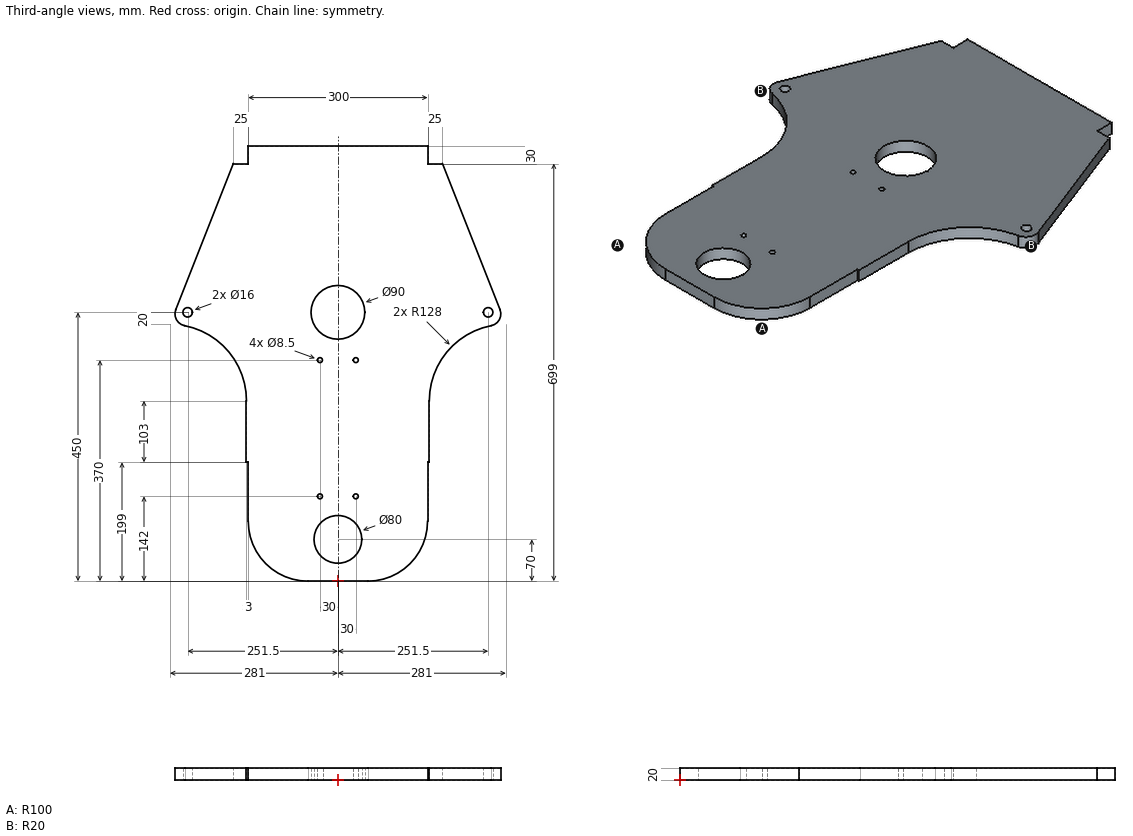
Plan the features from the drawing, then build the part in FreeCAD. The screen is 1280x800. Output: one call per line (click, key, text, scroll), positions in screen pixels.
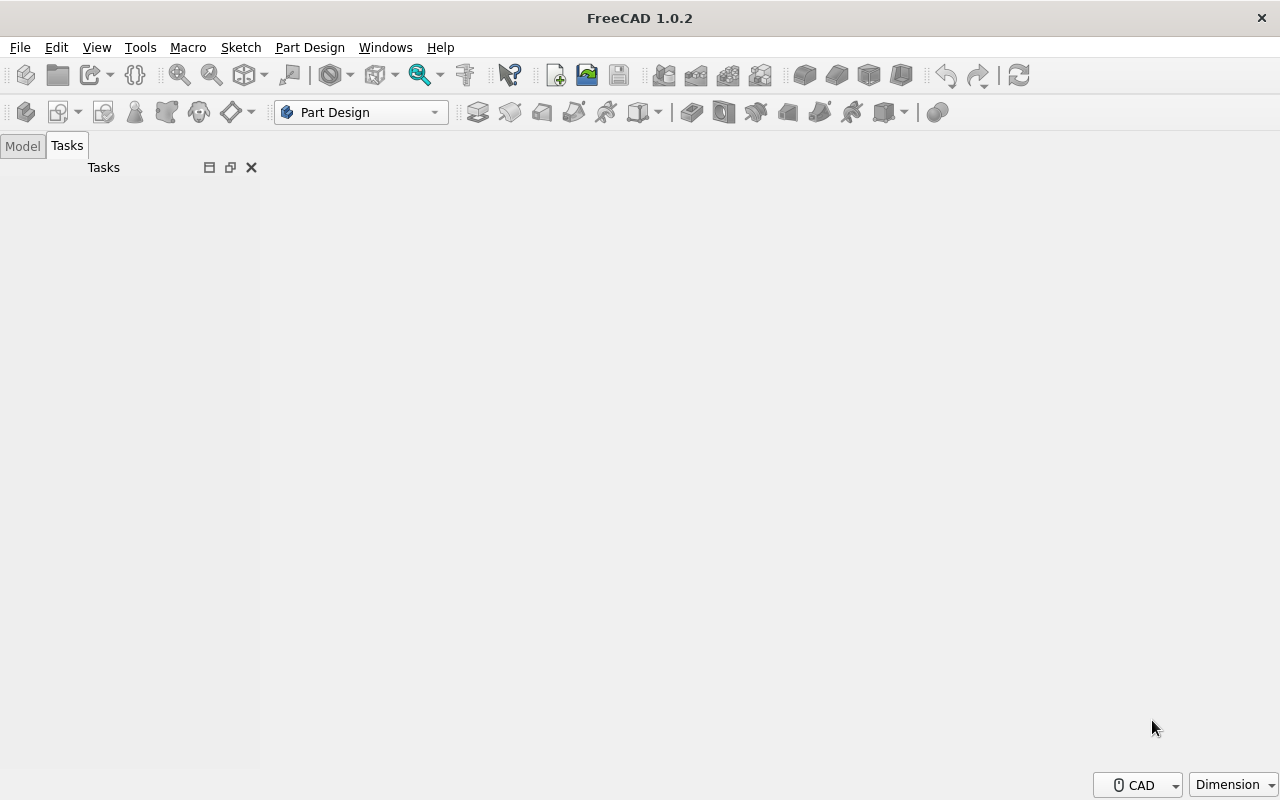
key(ctrl+n)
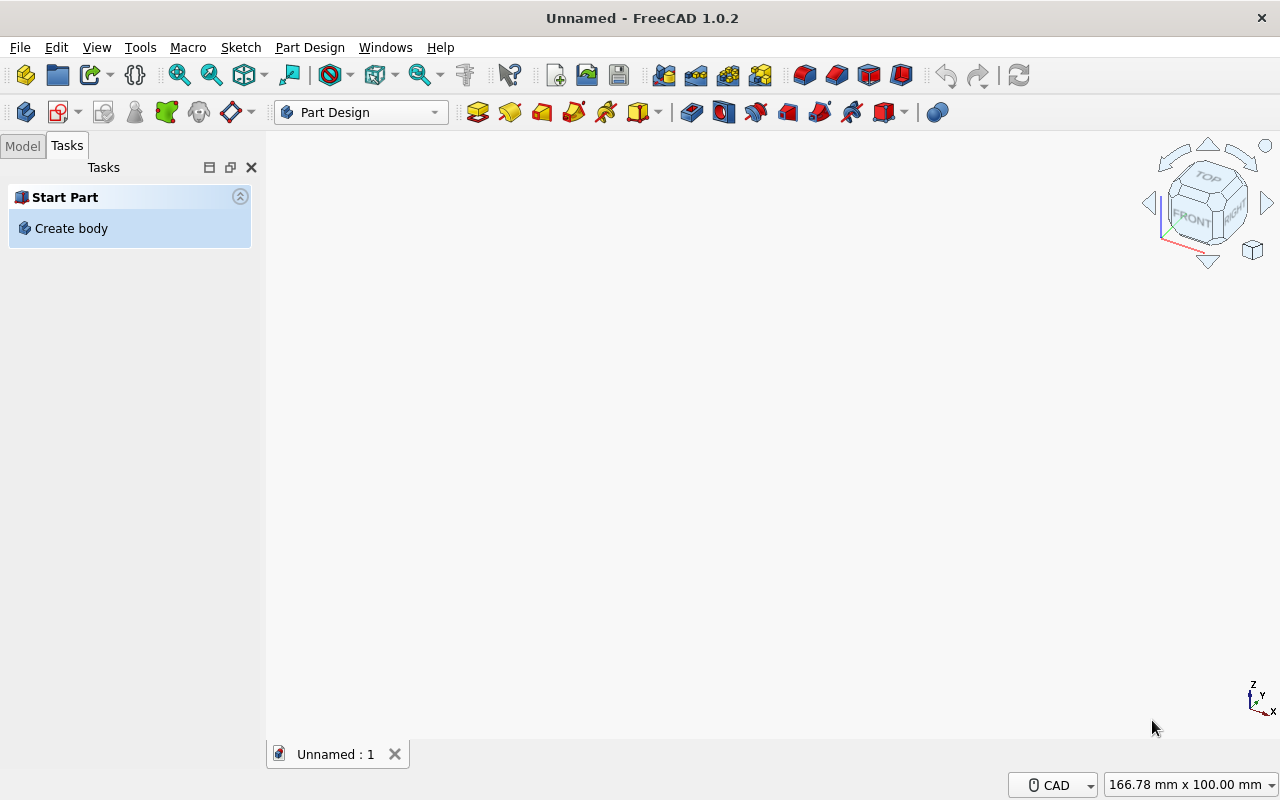
click(58, 112)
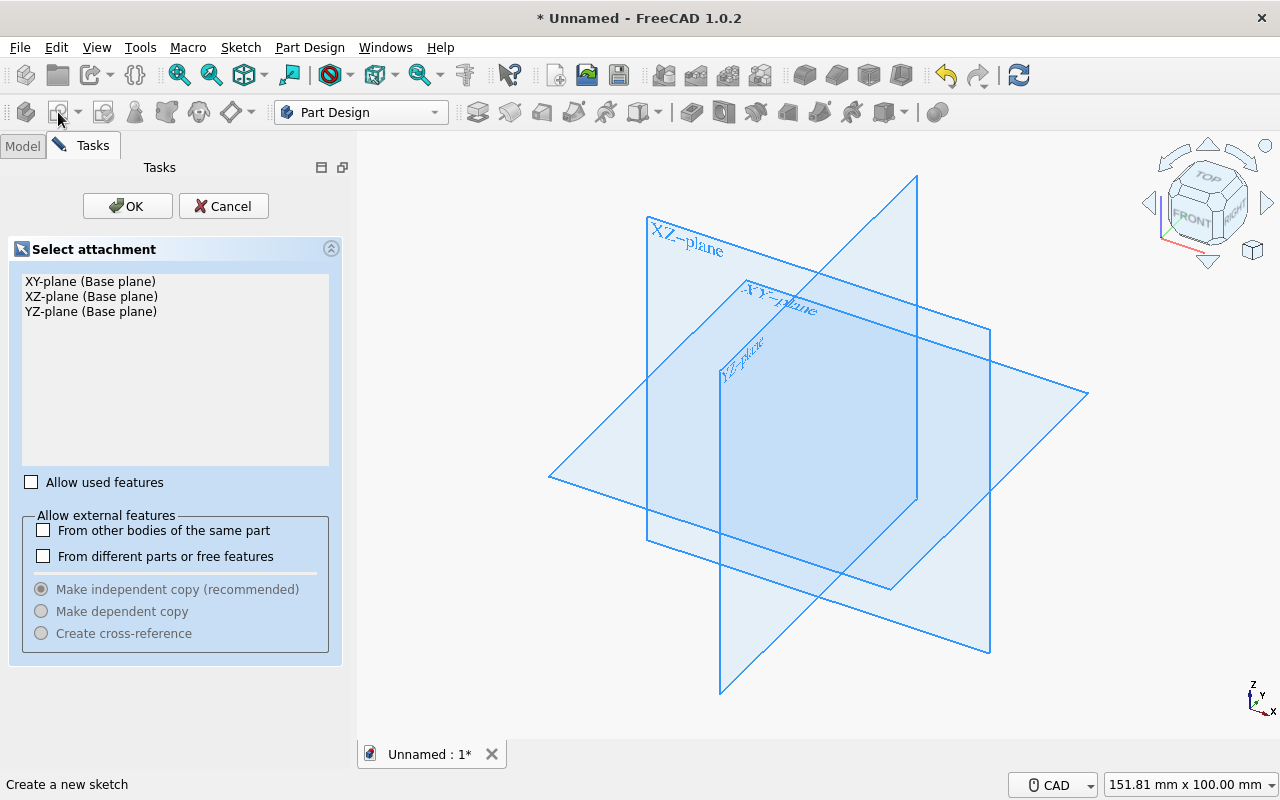
click(82, 282)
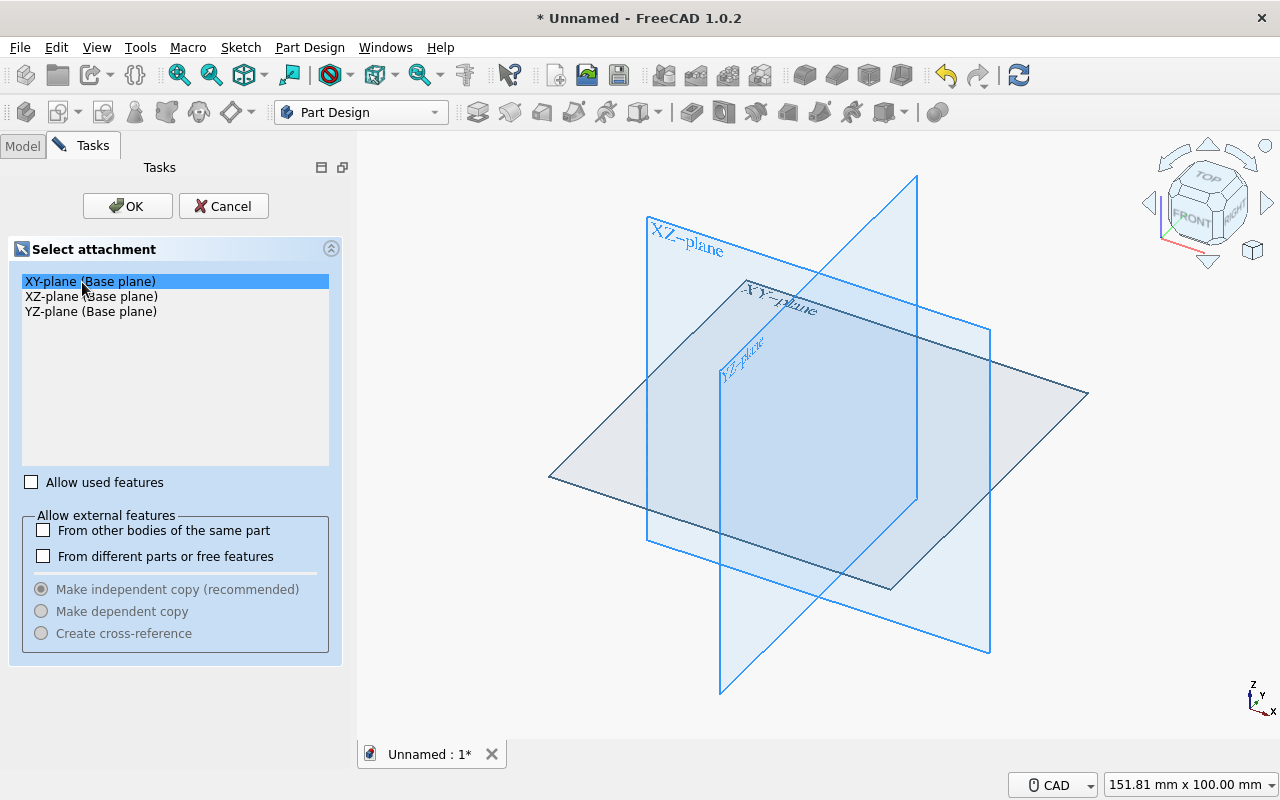
click(128, 206)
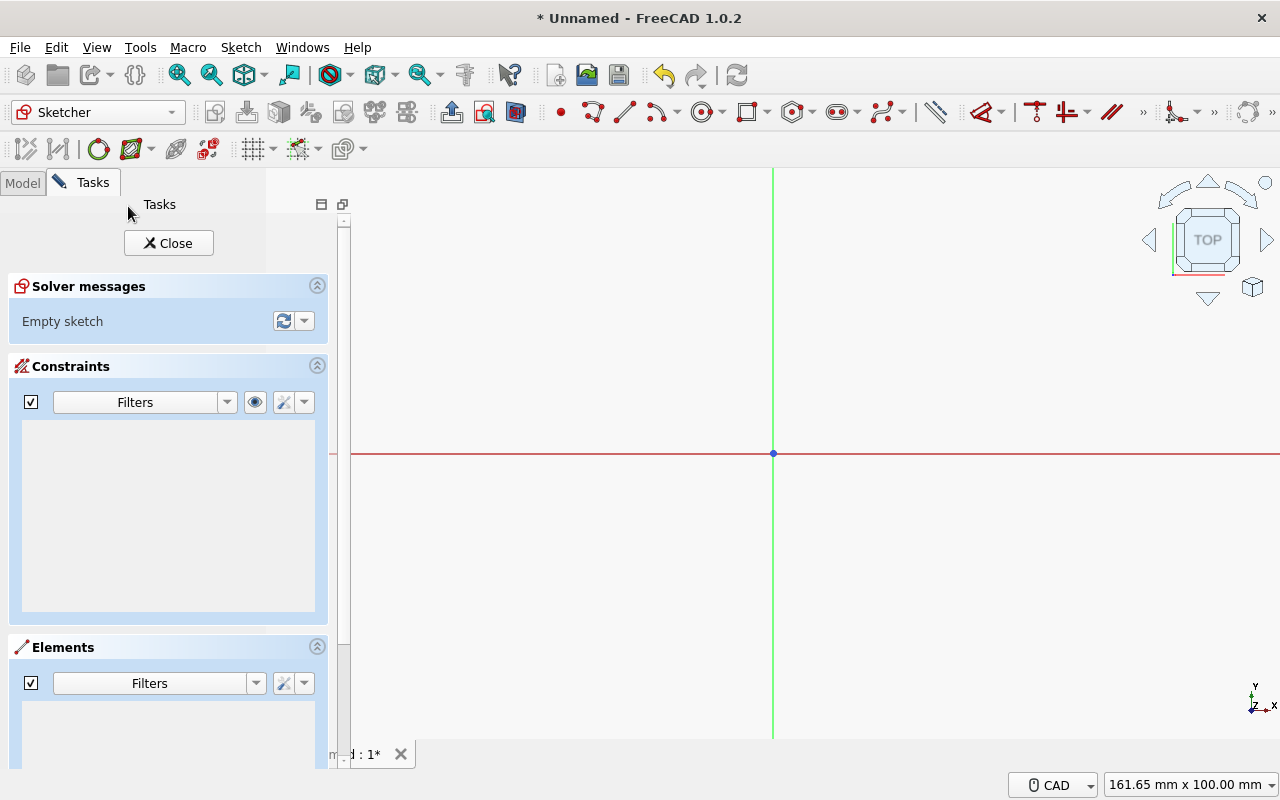
scroll(698, 661, down, 12)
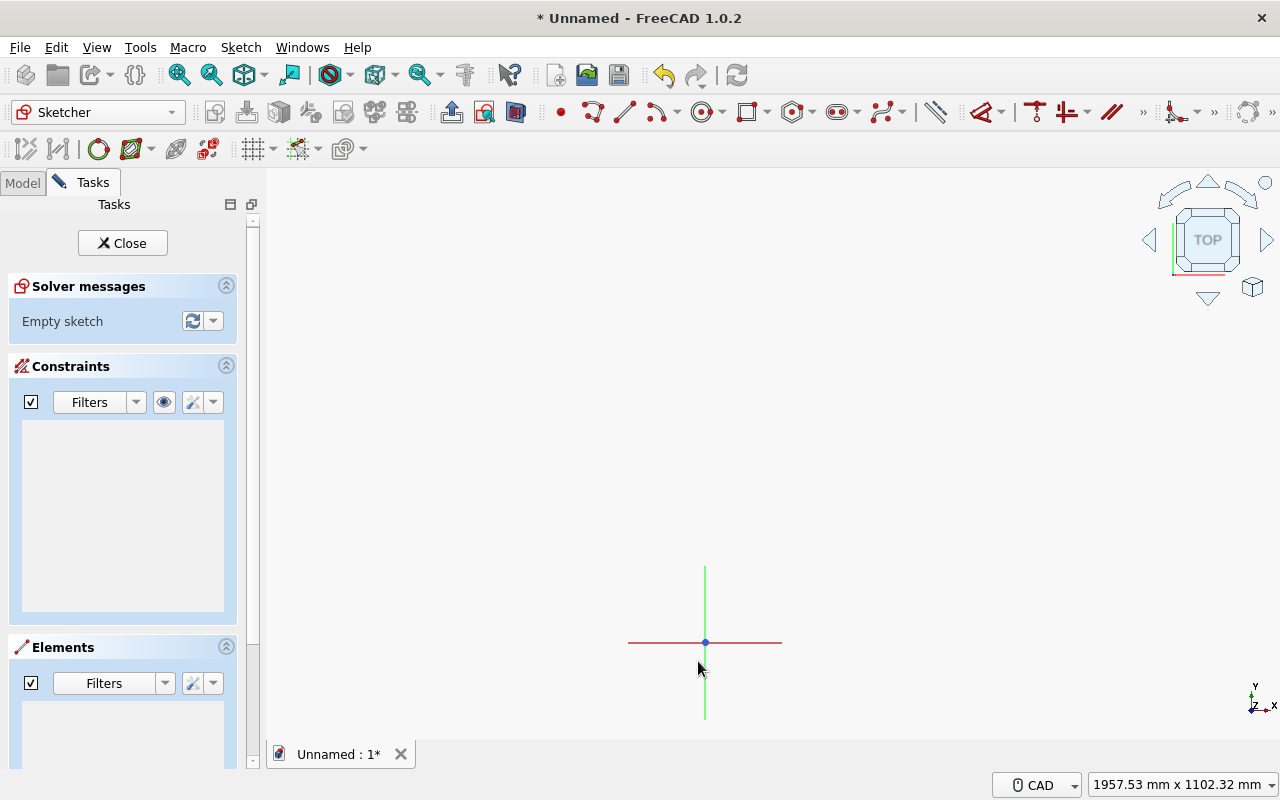
click(594, 112)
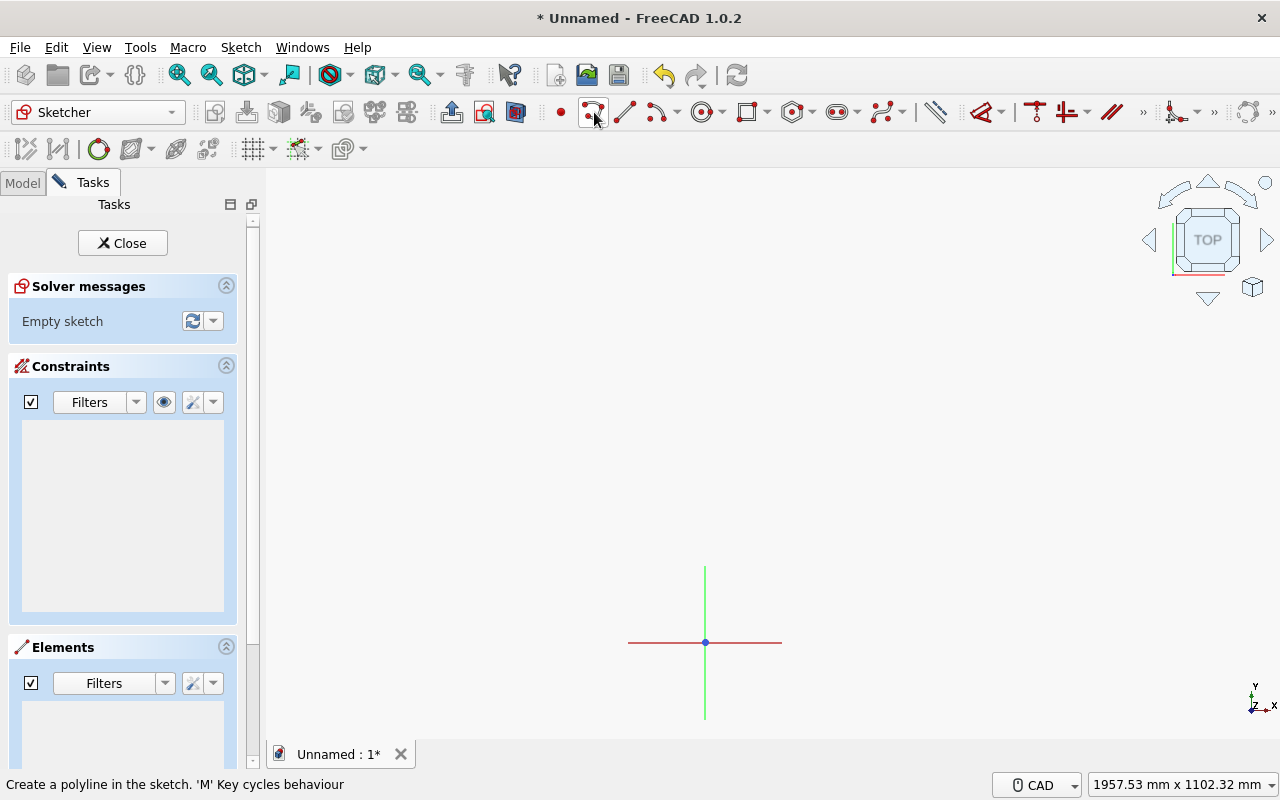
click(851, 420)
click(796, 281)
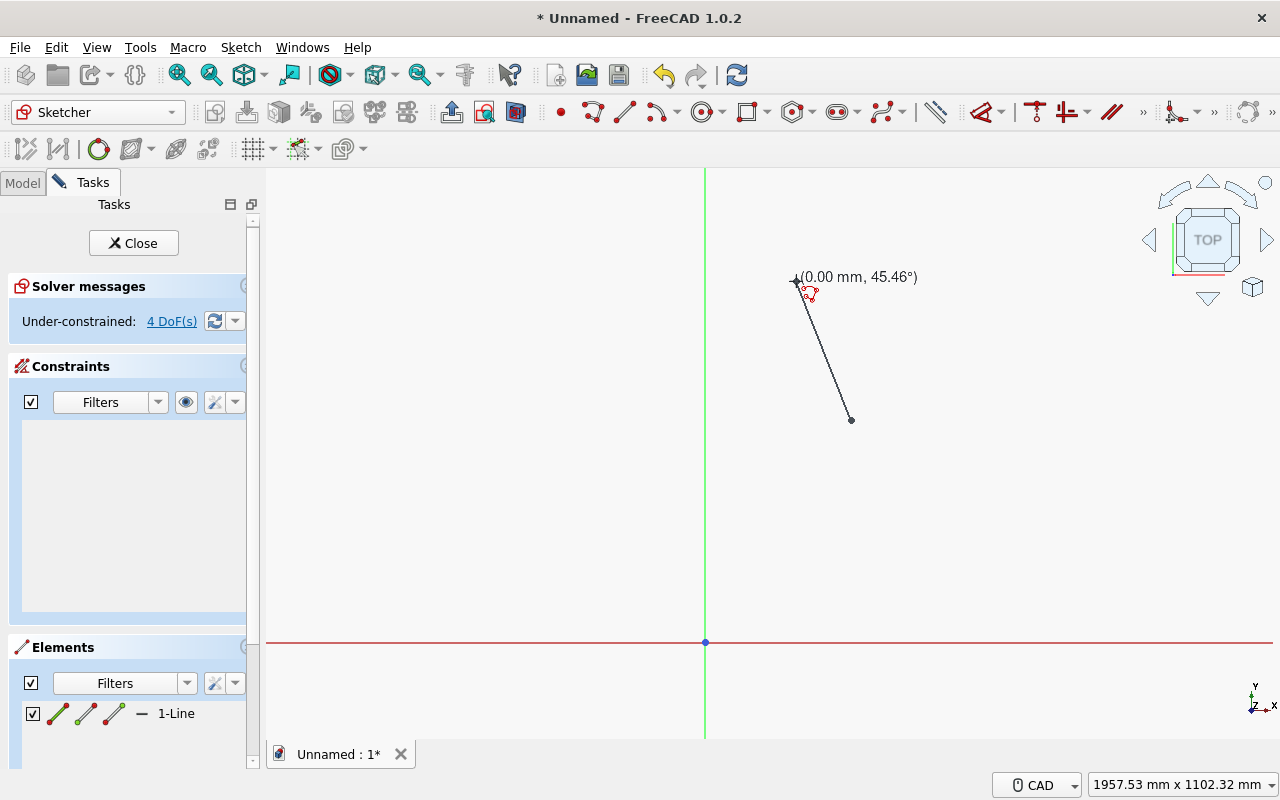
scroll(783, 281, up, 2)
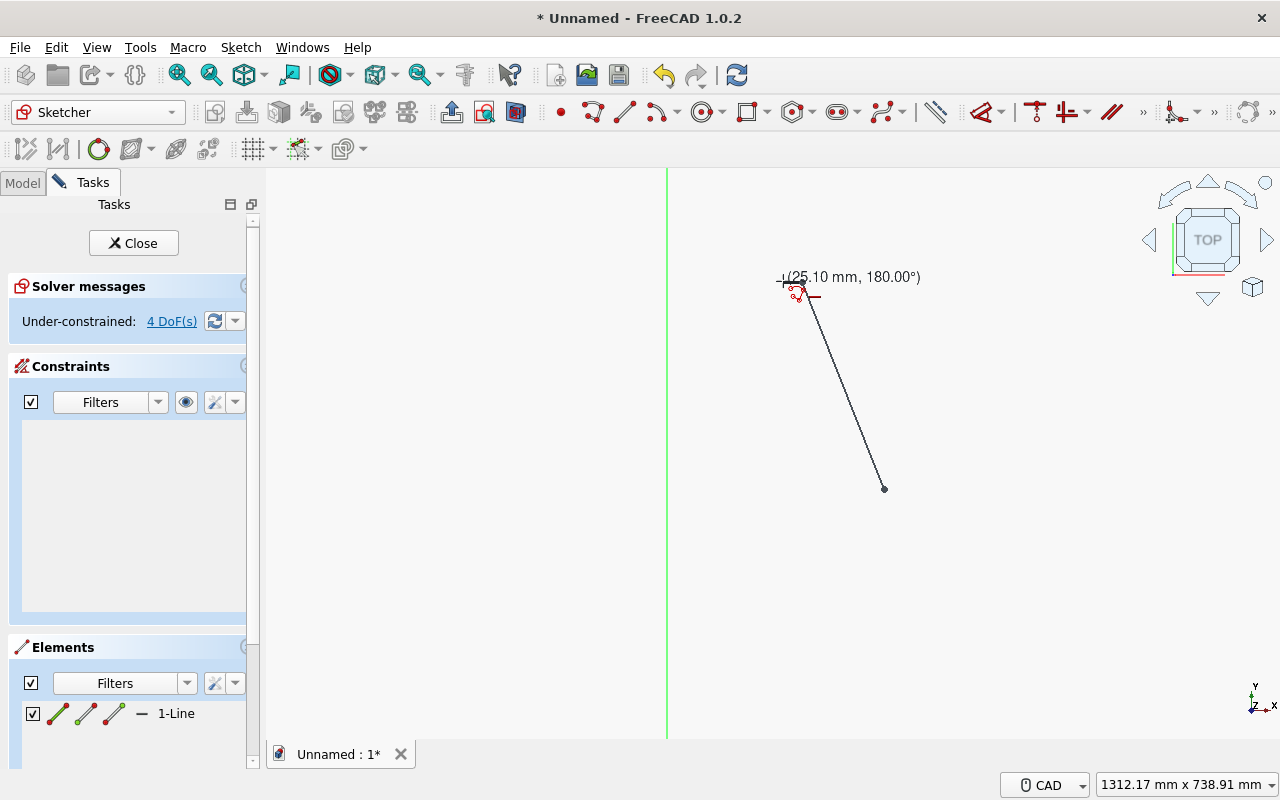
click(783, 281)
click(783, 258)
click(551, 258)
click(551, 281)
click(531, 281)
click(450, 489)
right_click(450, 489)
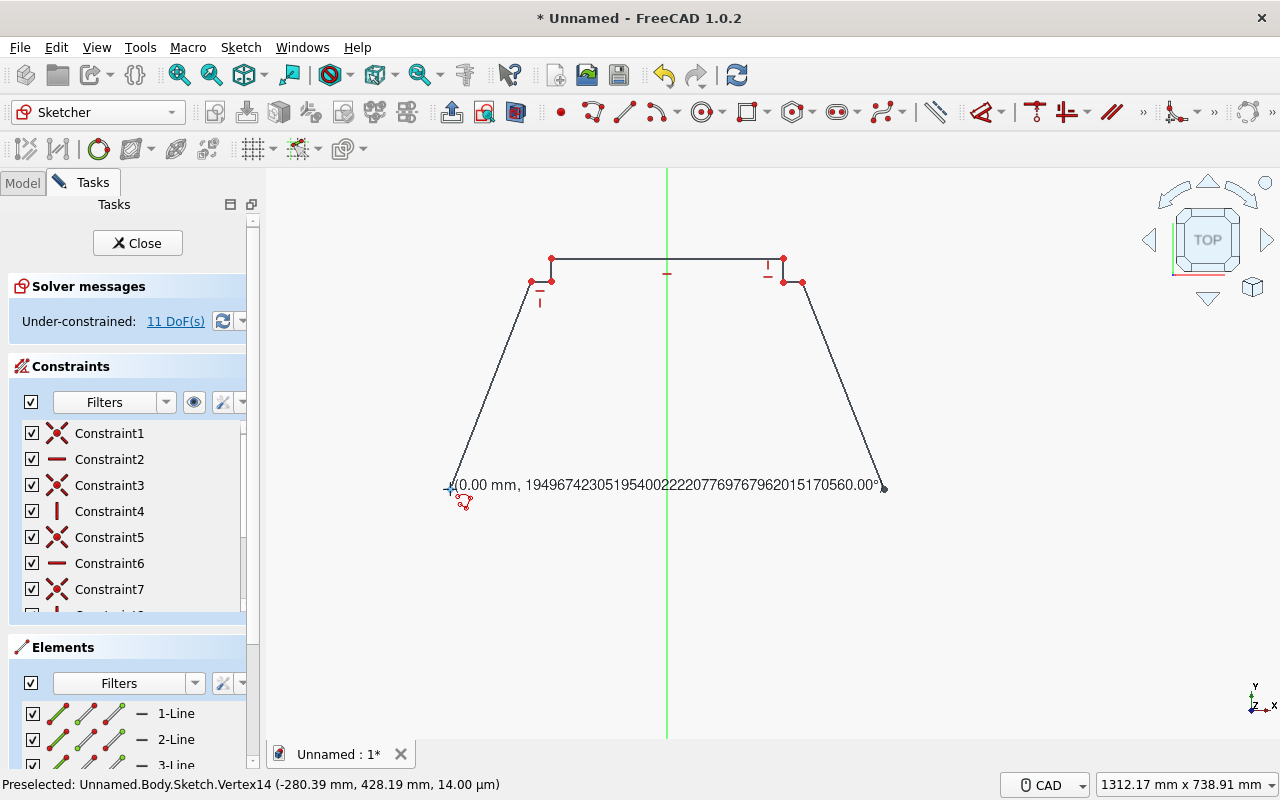
click(548, 588)
click(548, 667)